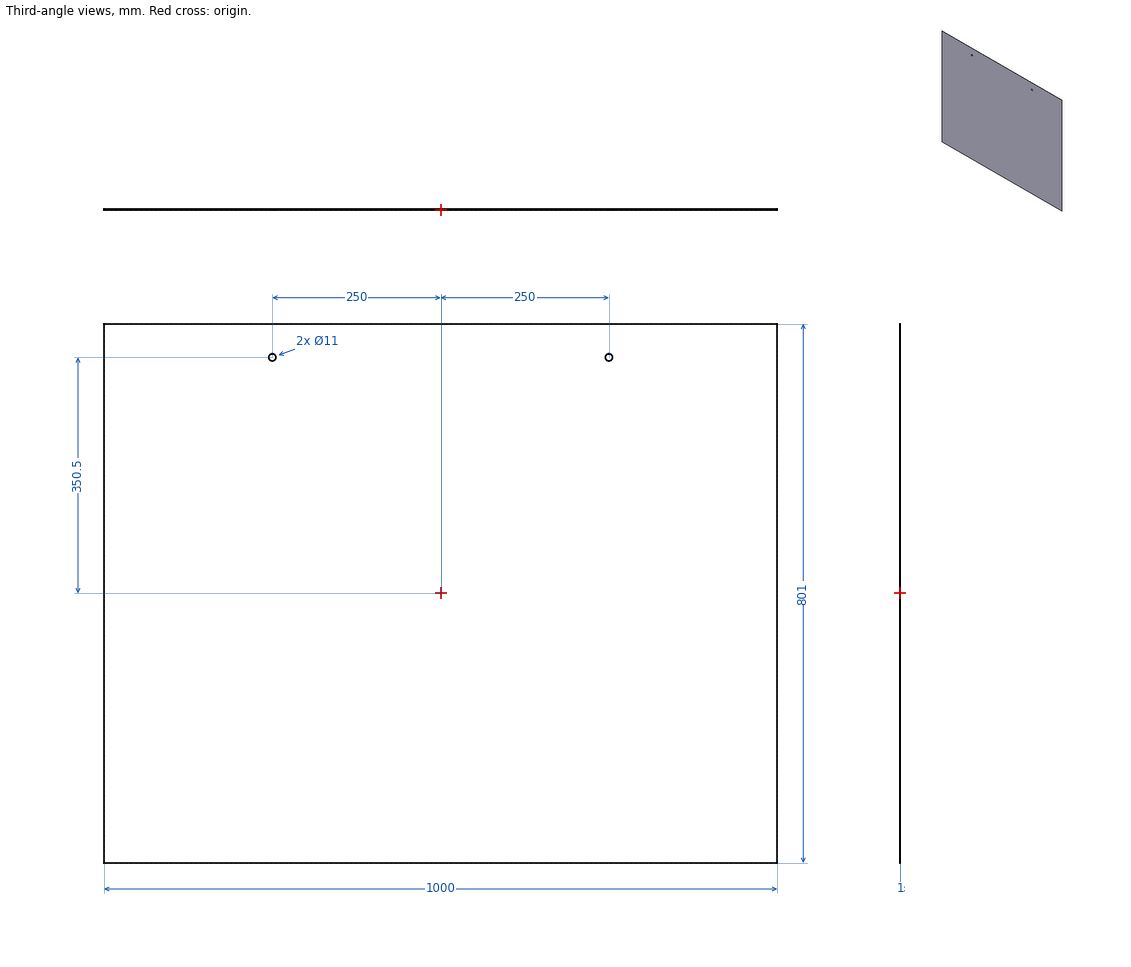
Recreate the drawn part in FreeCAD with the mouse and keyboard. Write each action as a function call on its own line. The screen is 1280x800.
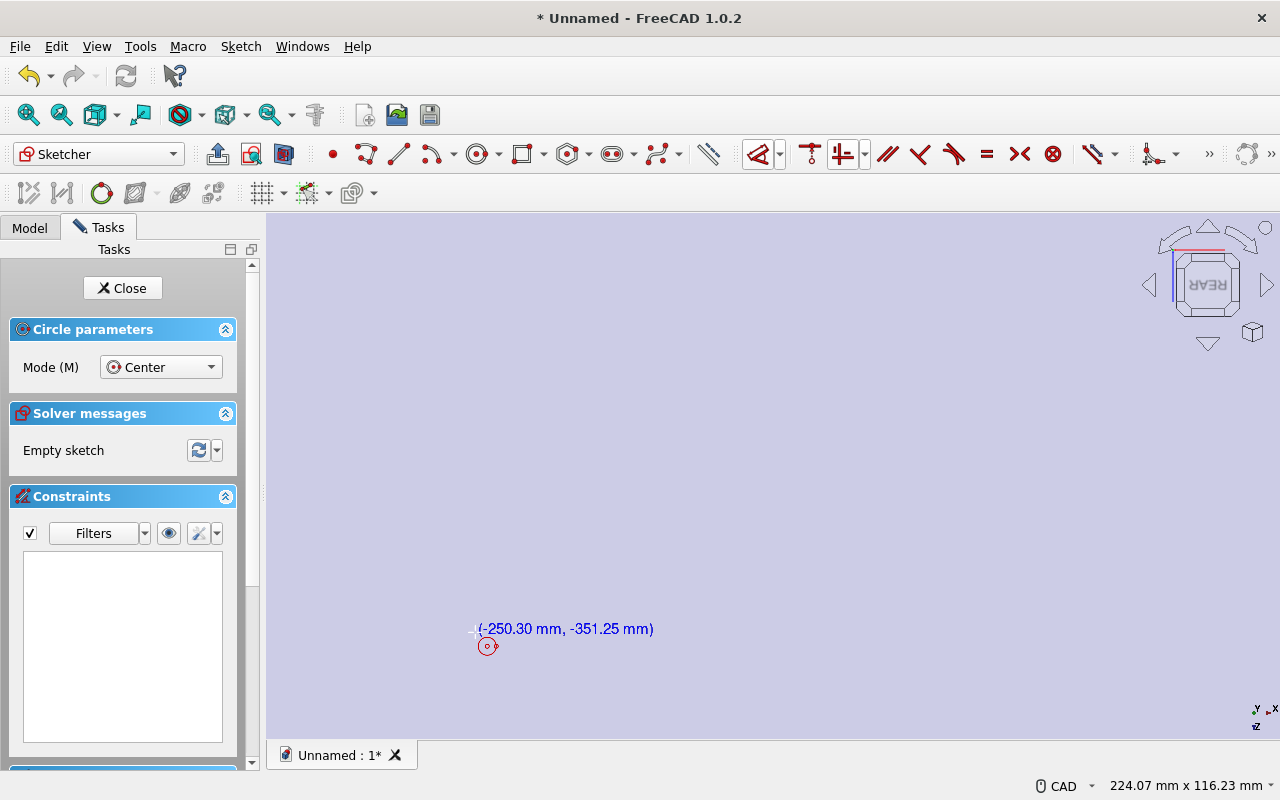
scroll(476, 634, down, 8)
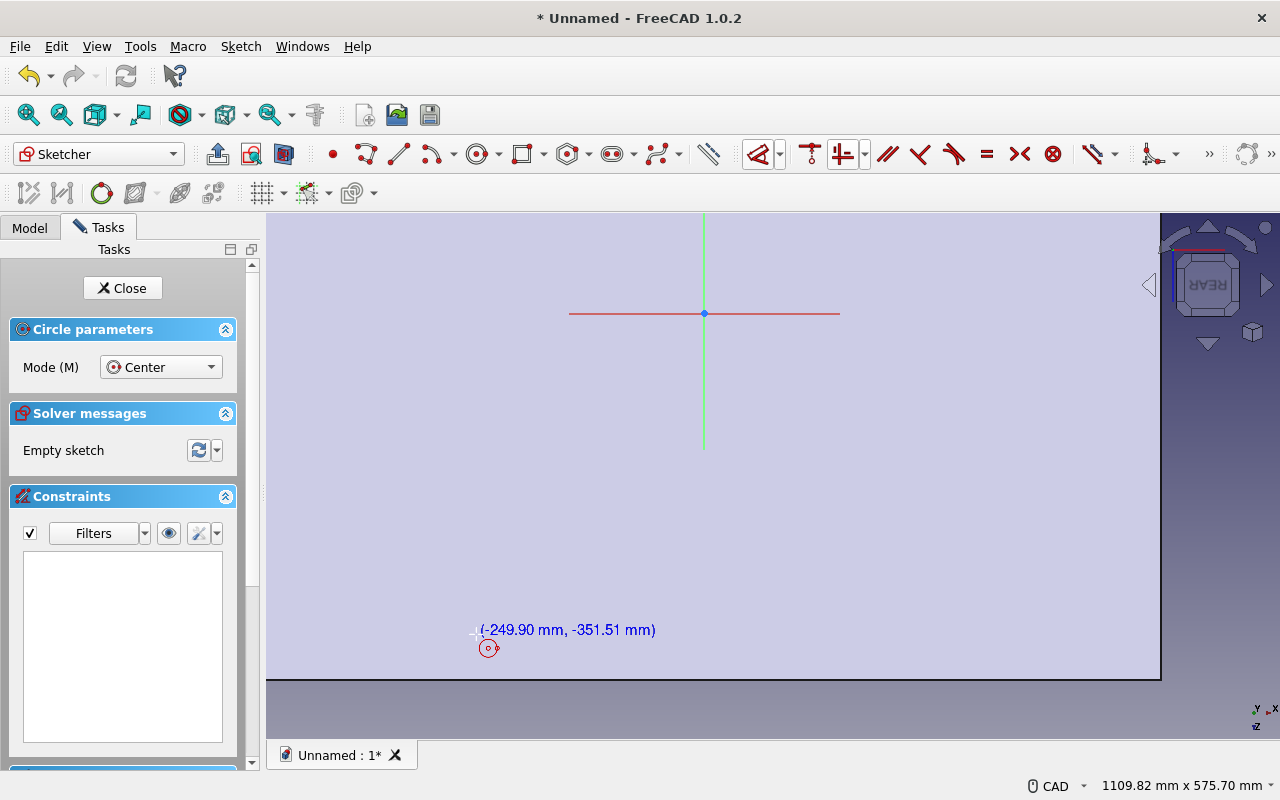
click(476, 634)
move(480, 630)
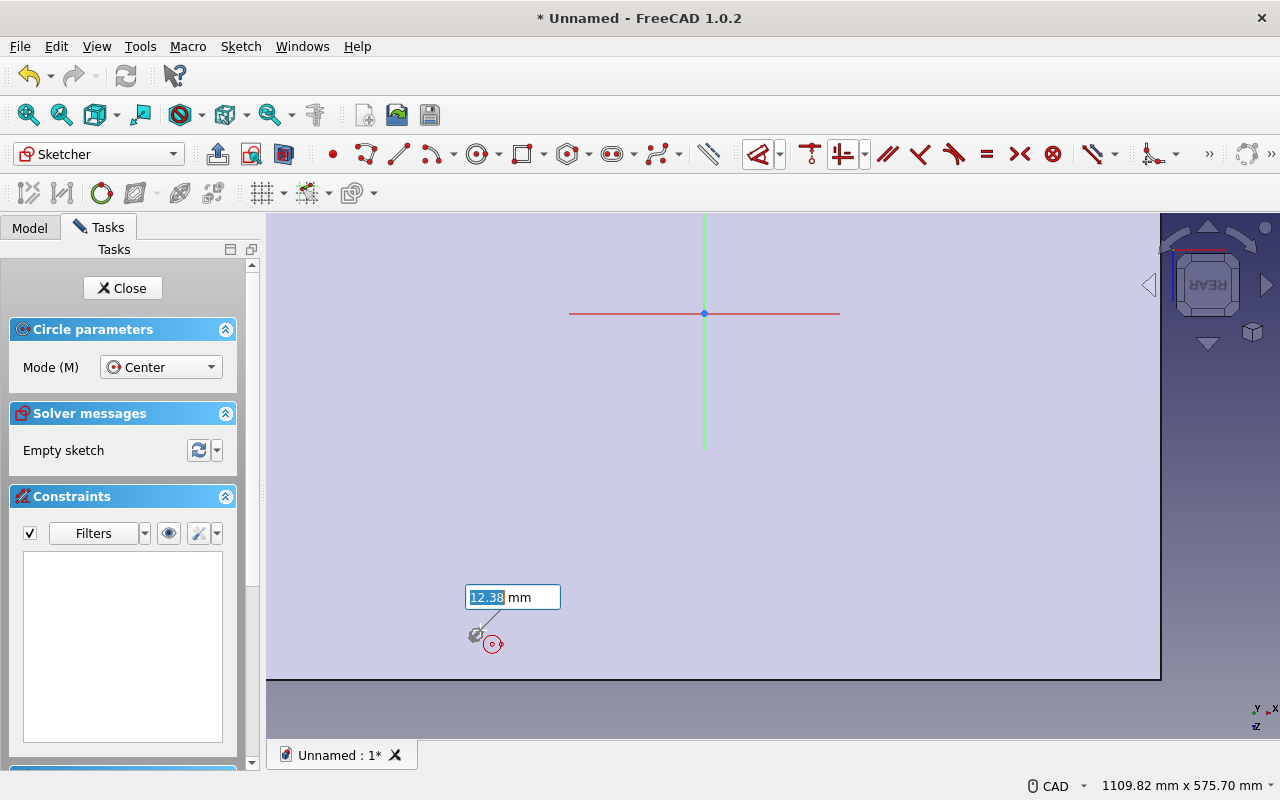
text(11)
key(Return)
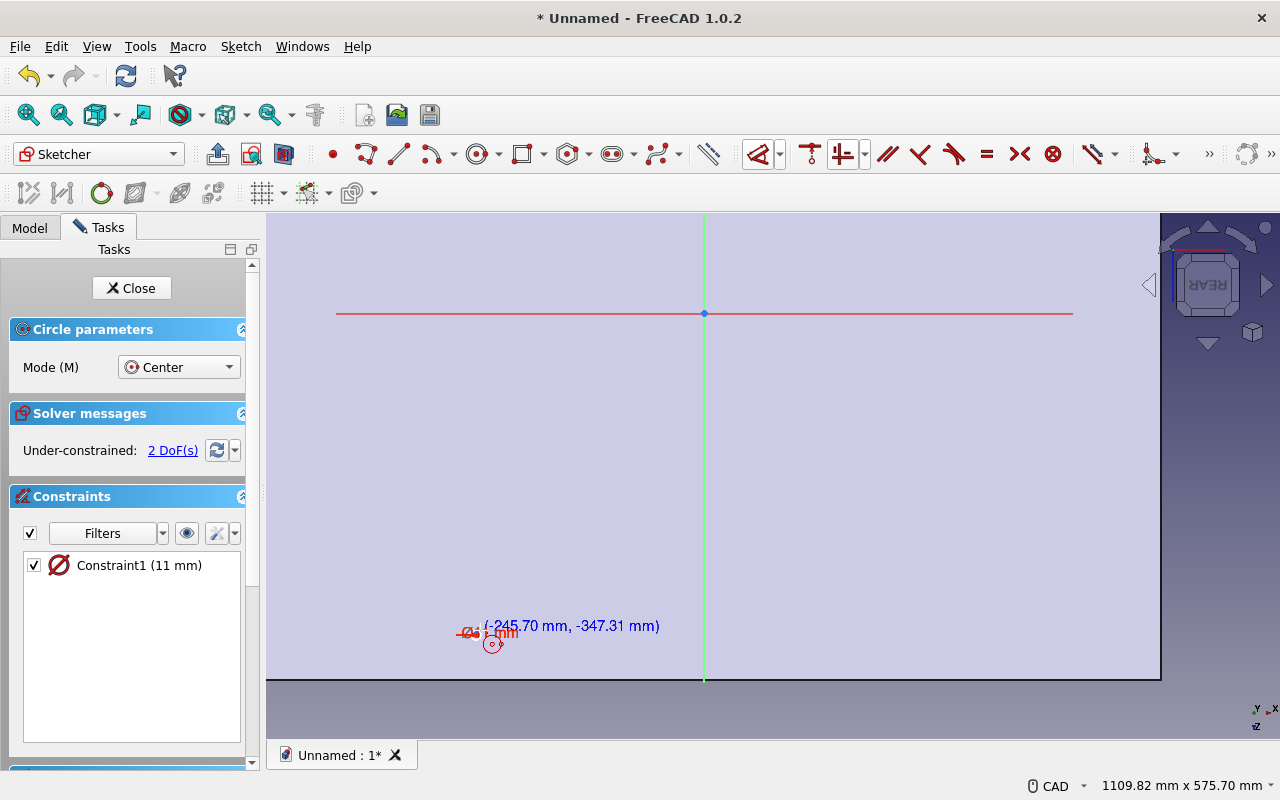
scroll(933, 634, up, 8)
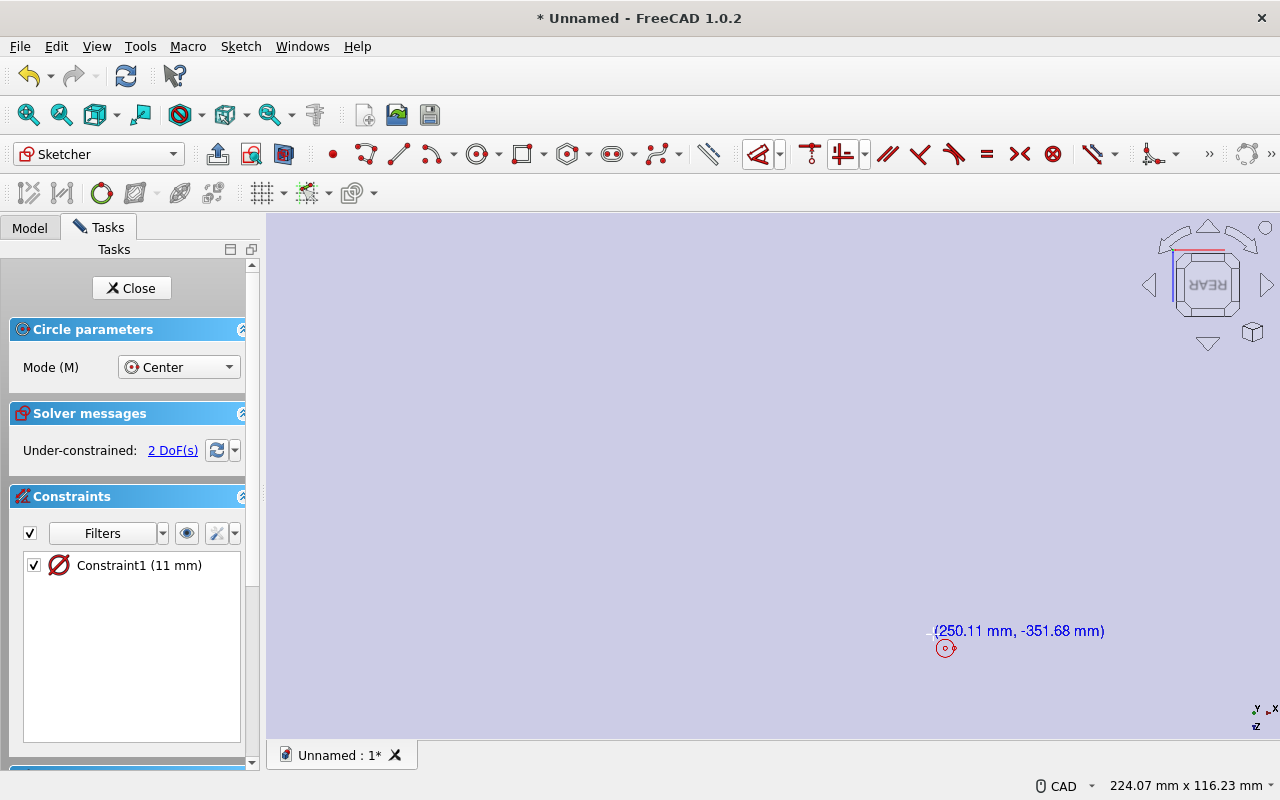
scroll(934, 634, down, 8)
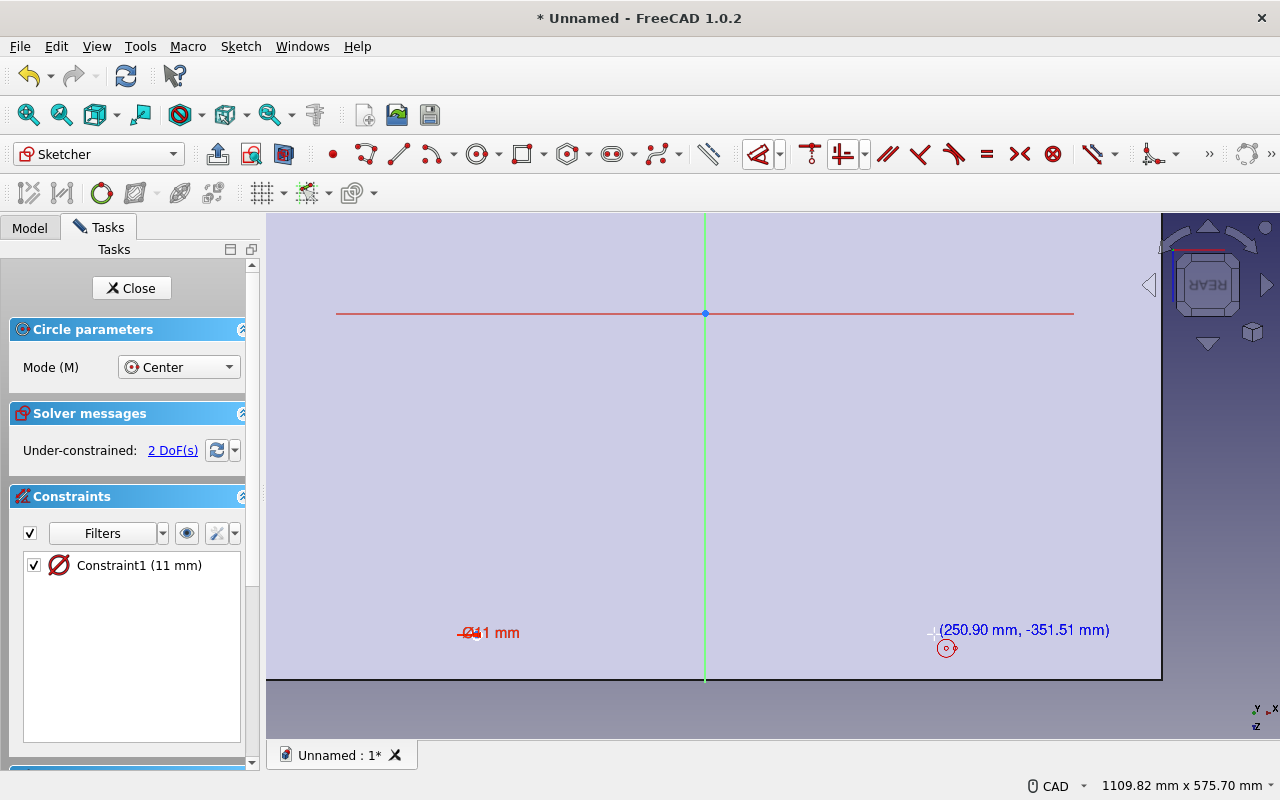
click(934, 634)
move(937, 630)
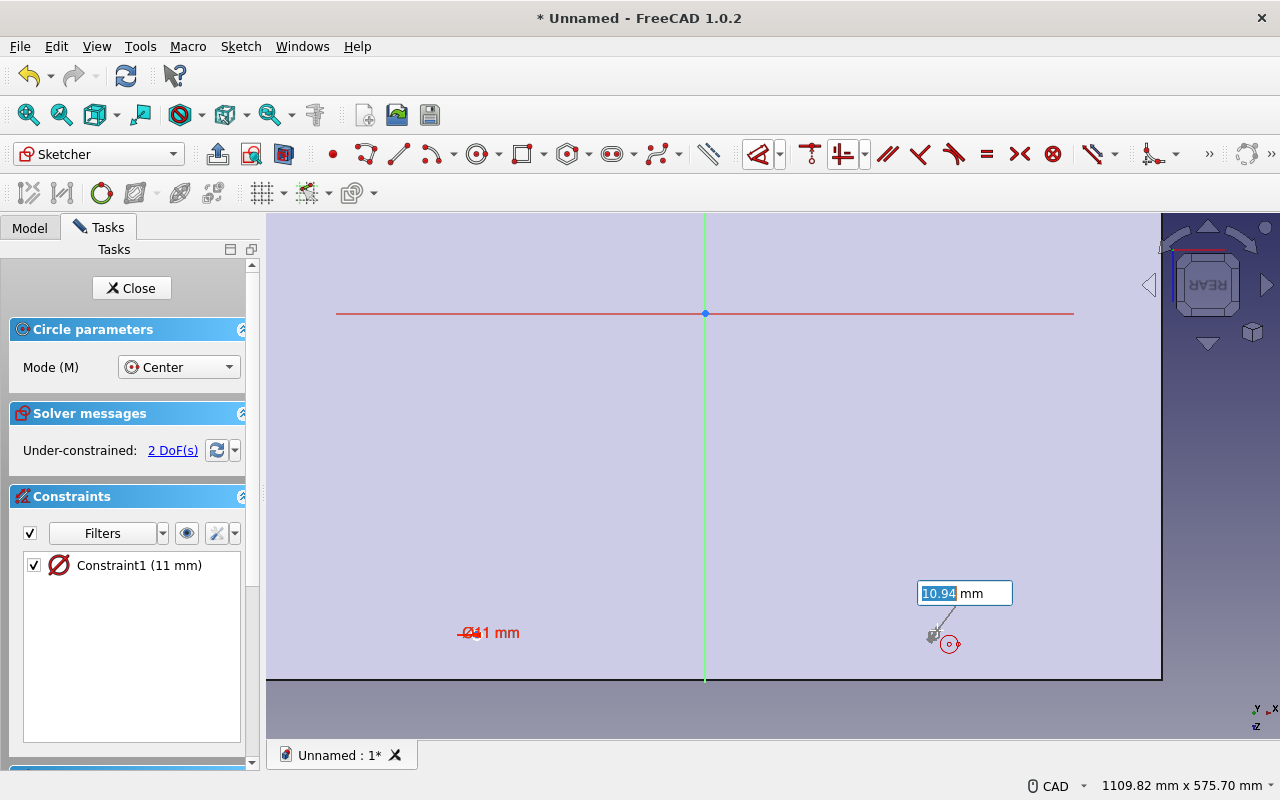
text(11)
key(Return)
key(Escape)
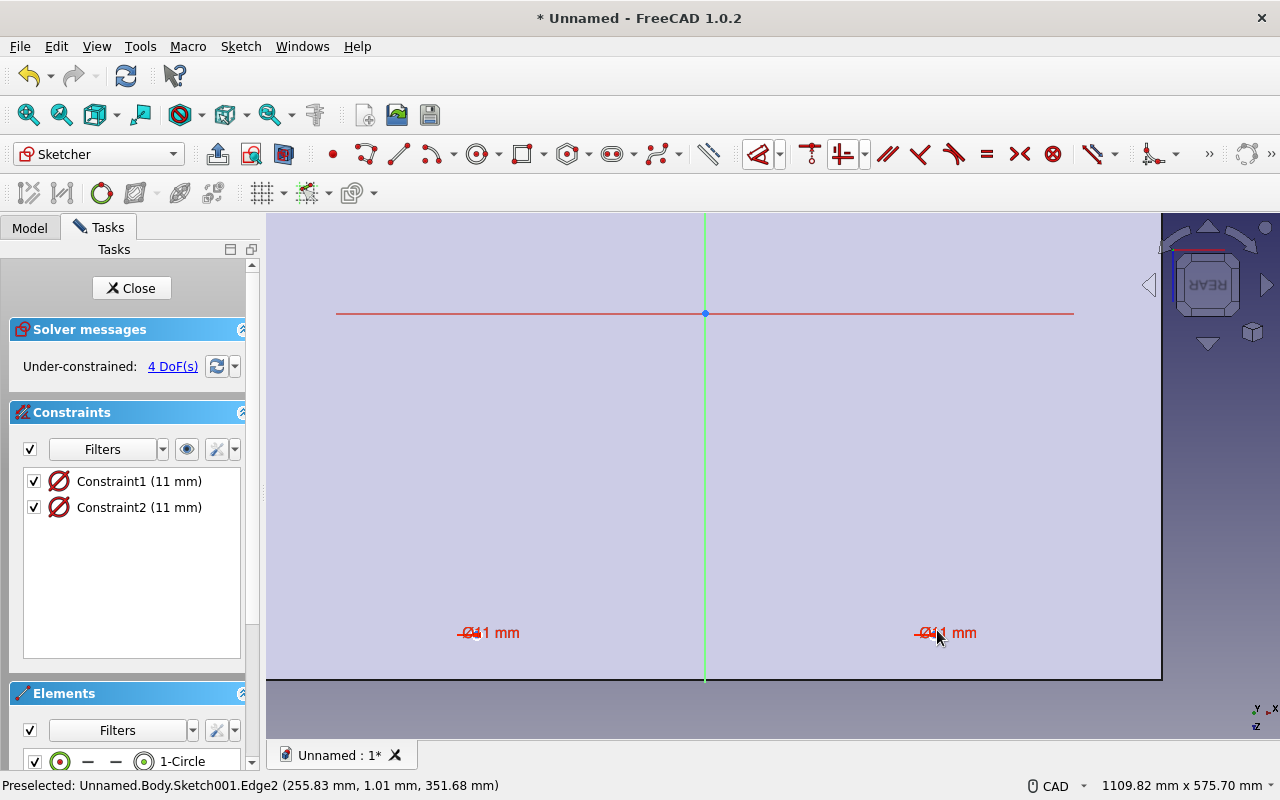
click(477, 635)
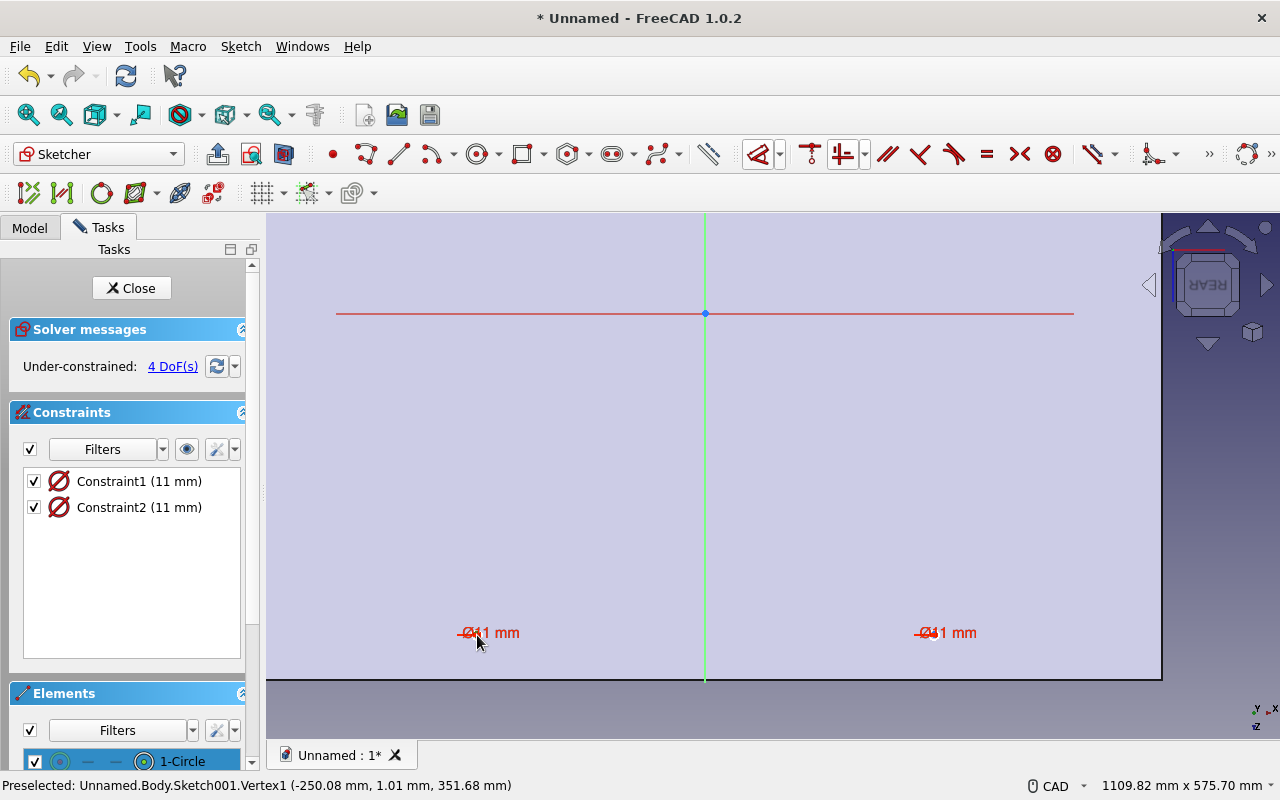
click(934, 635)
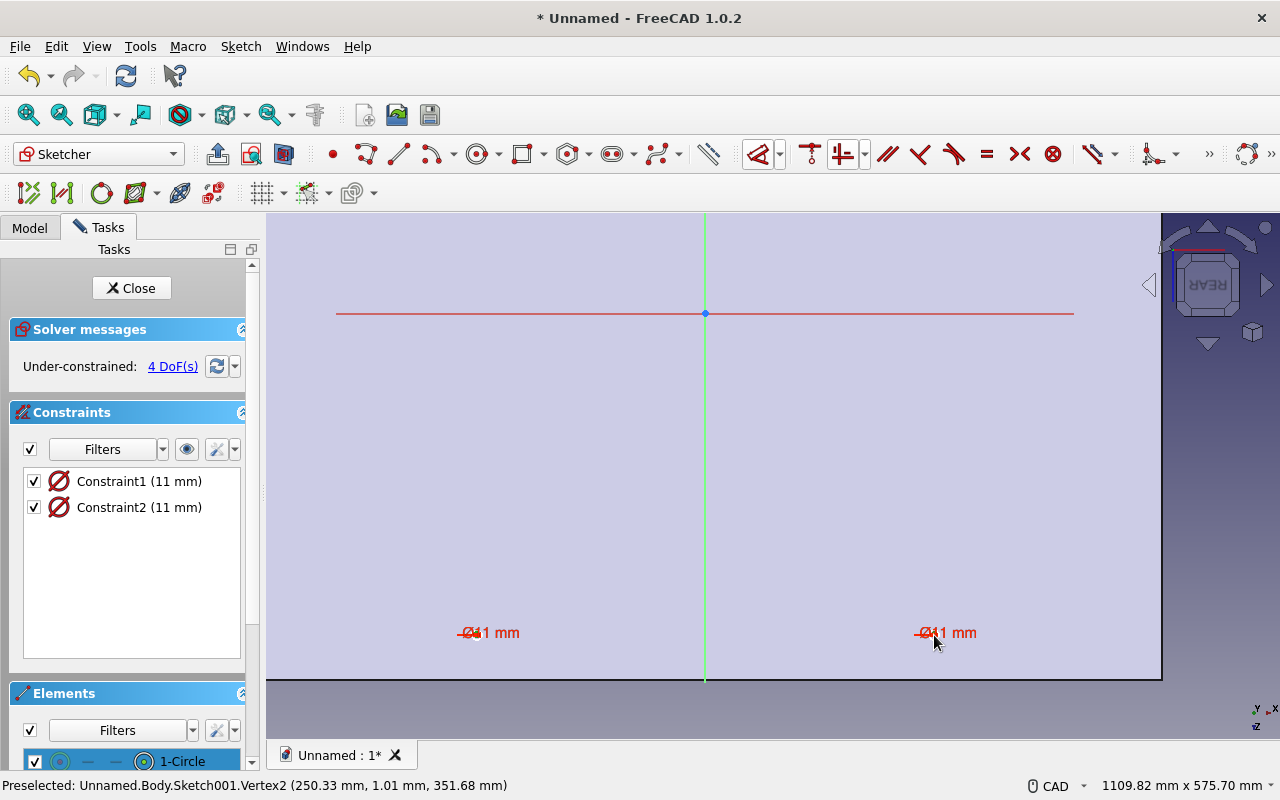
key(h)